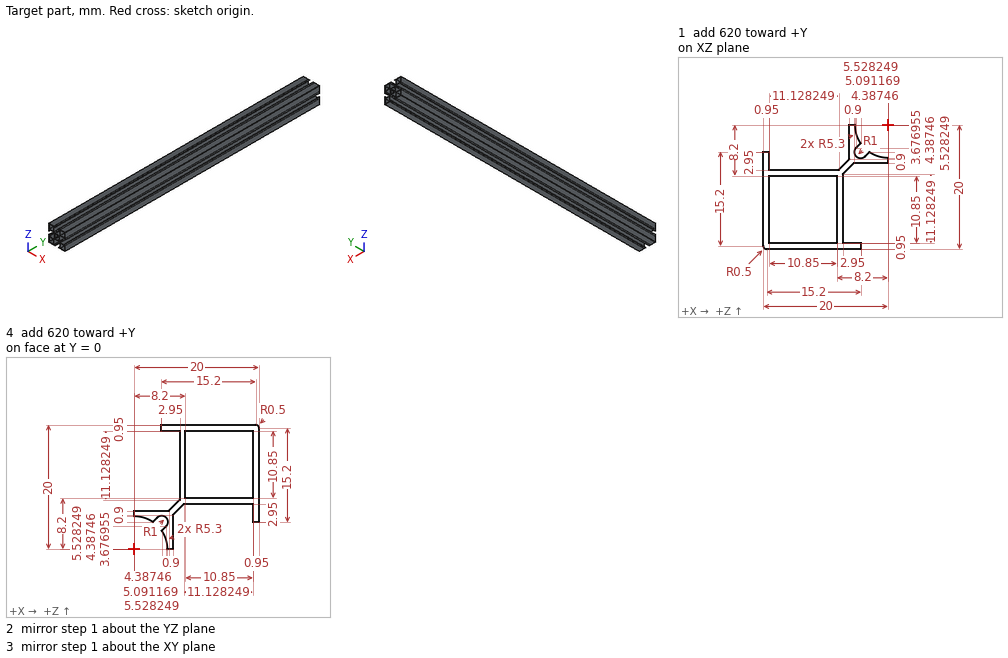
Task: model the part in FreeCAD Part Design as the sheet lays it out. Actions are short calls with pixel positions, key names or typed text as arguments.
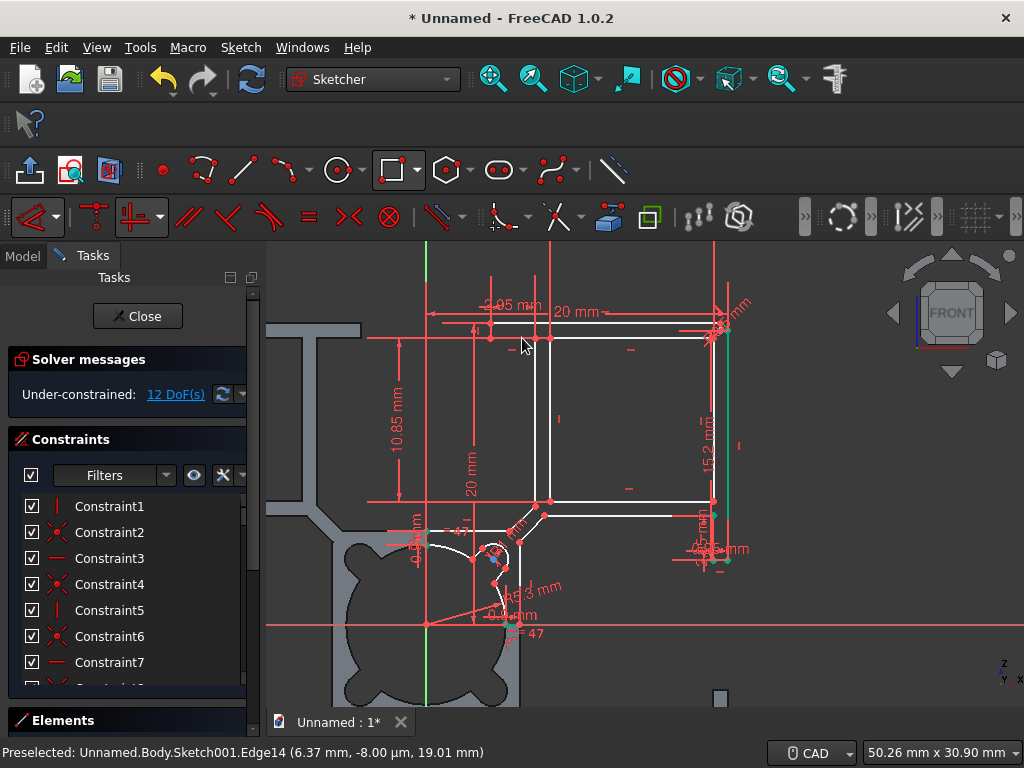
scroll(491, 331, up, 6)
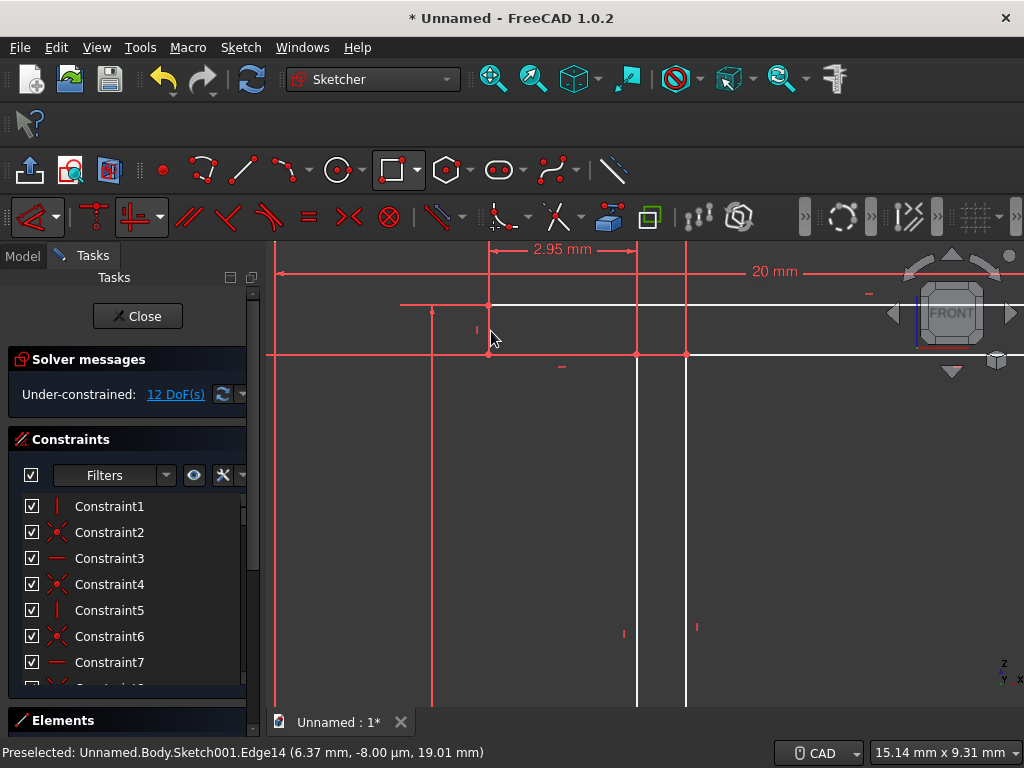
click(489, 330)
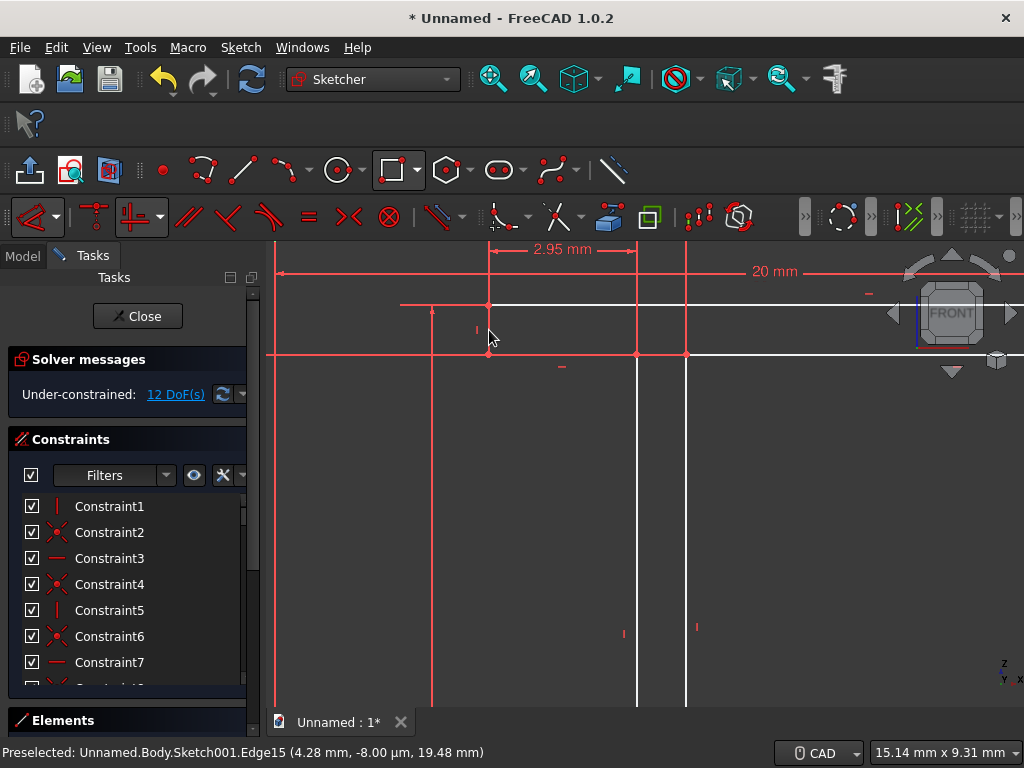
click(58, 218)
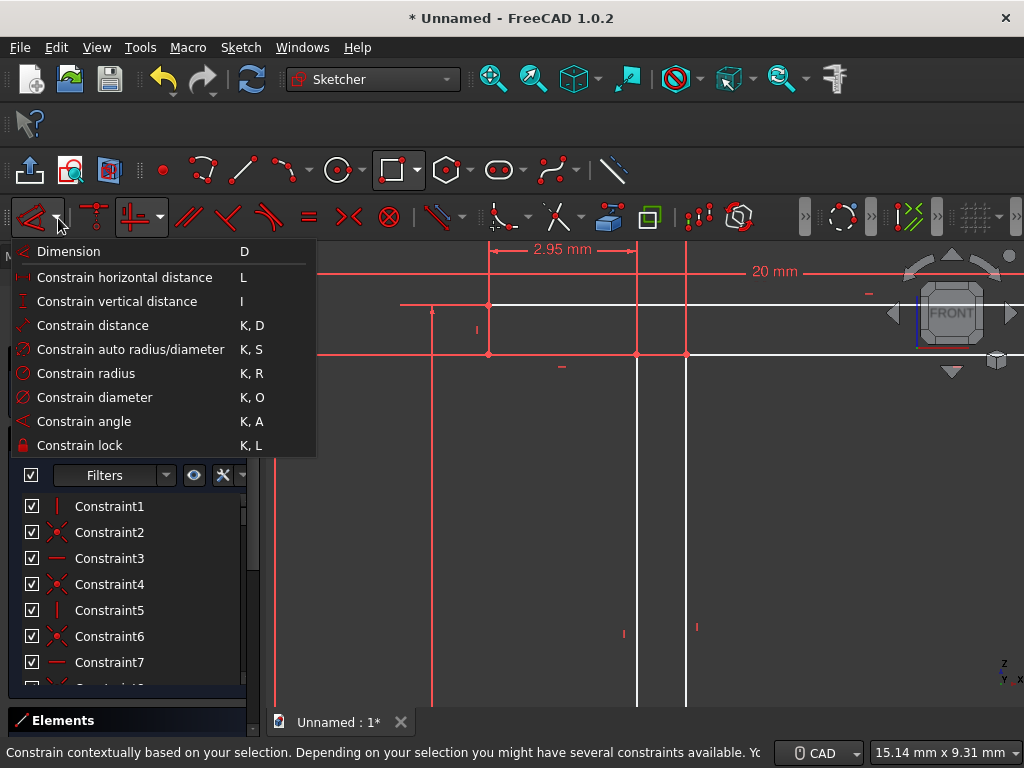
click(164, 301)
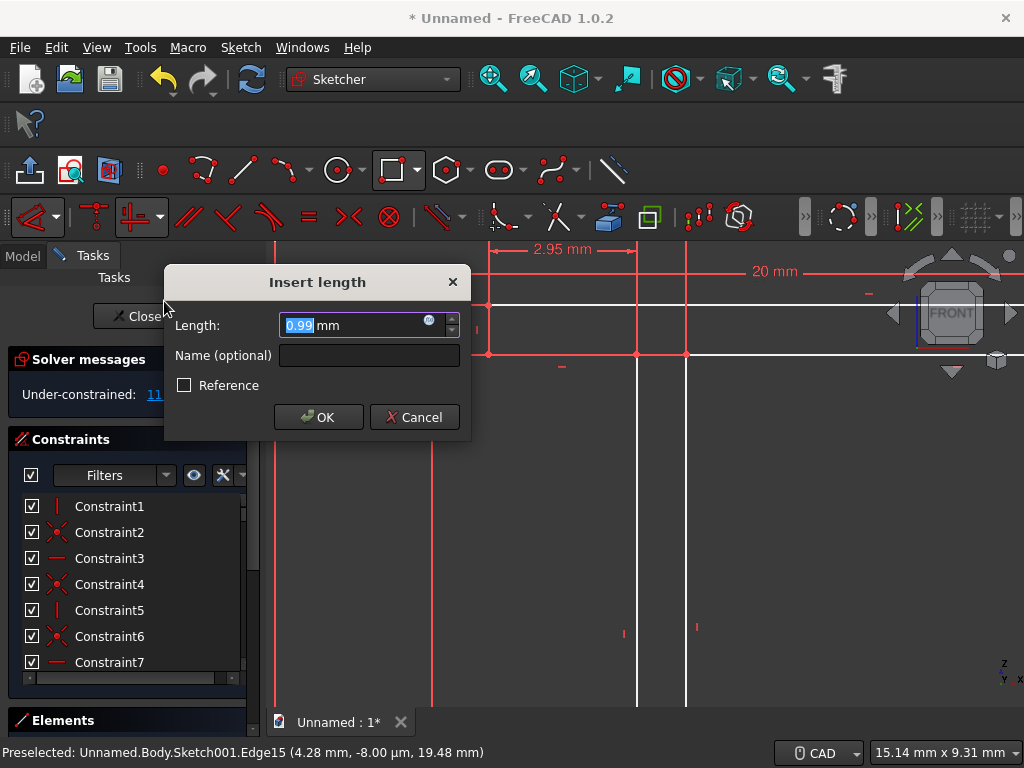
text(0.95)
key(Return)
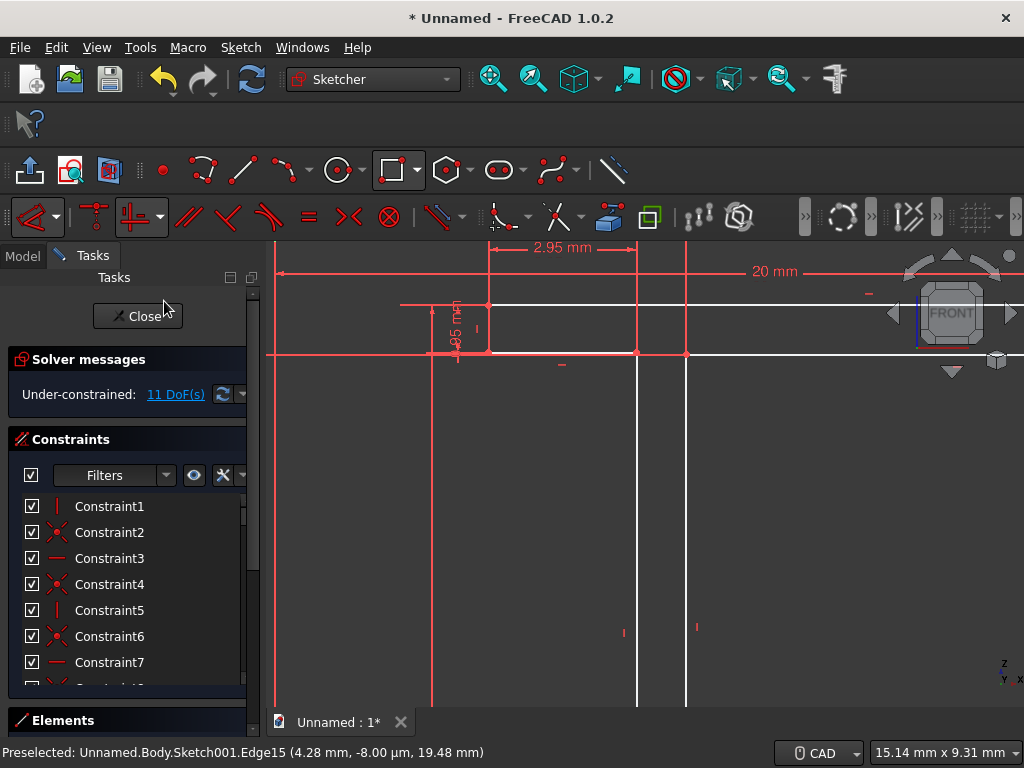
click(717, 305)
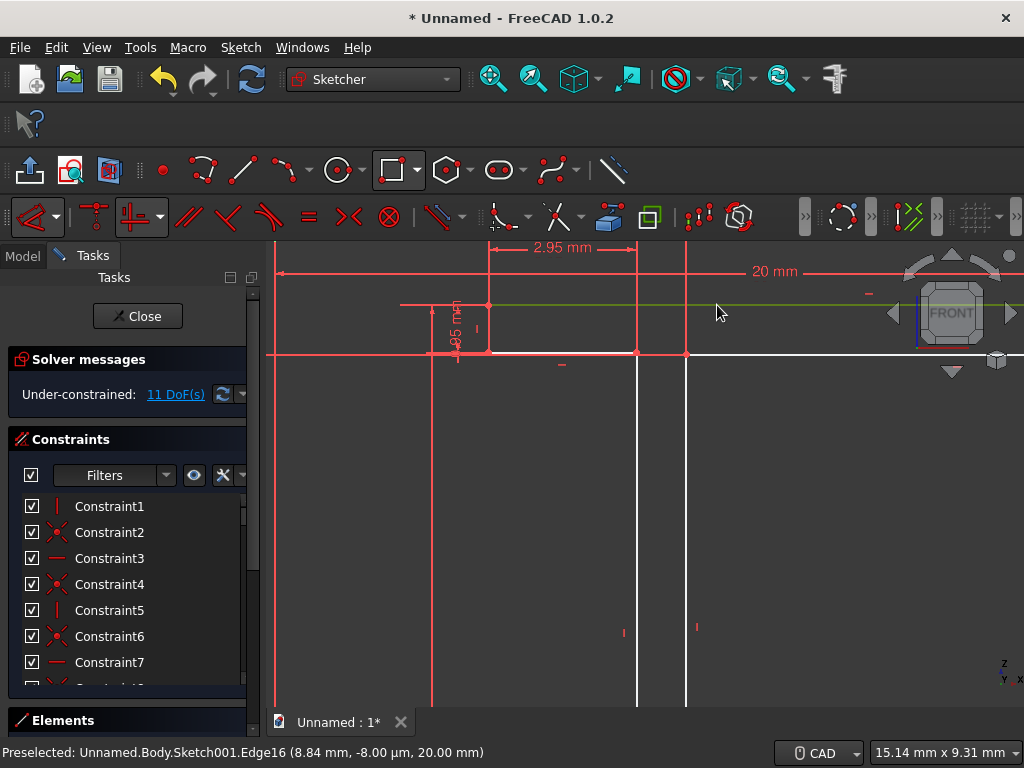
key(l)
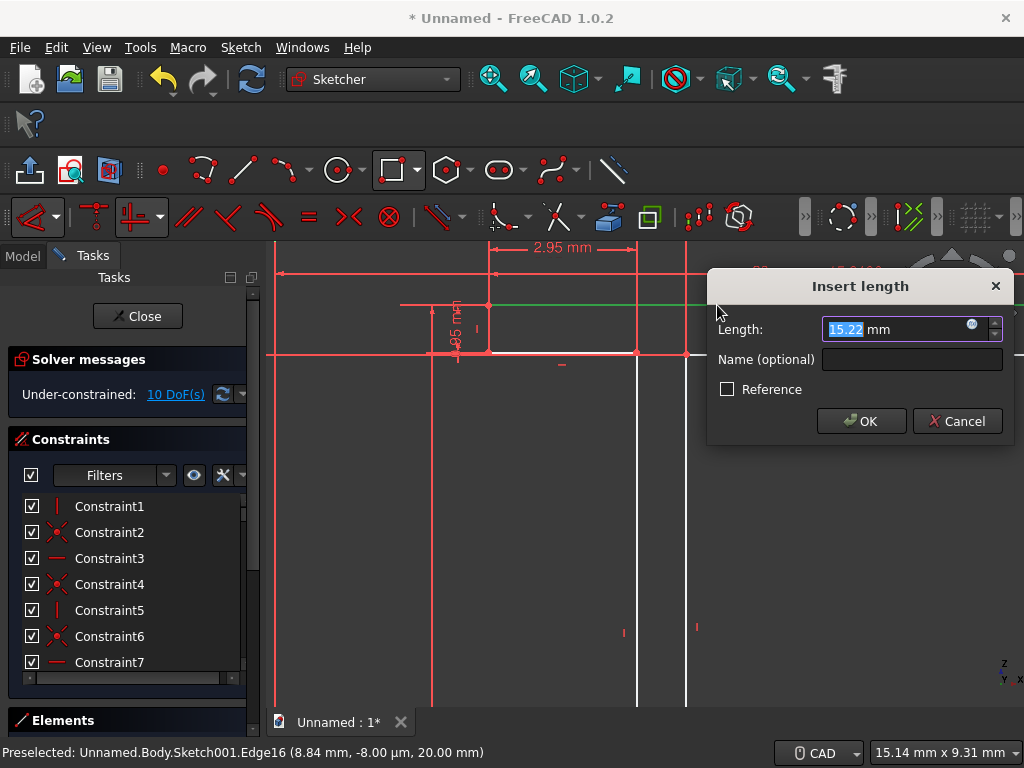
text(15.2)
key(Return)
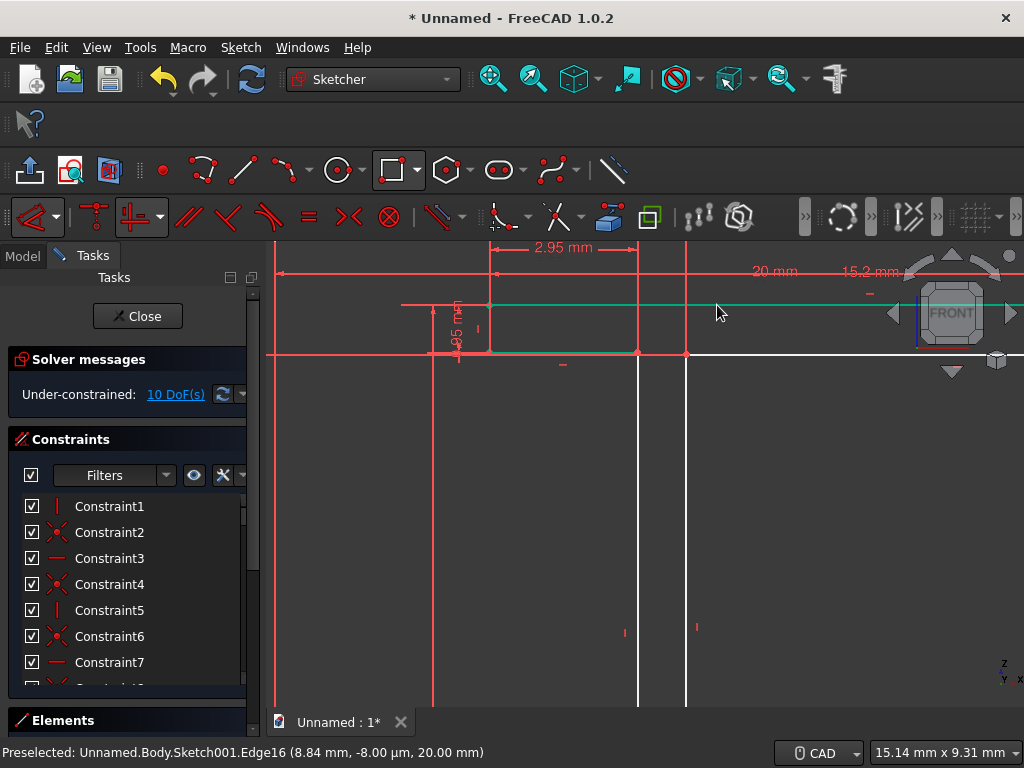
click(686, 355)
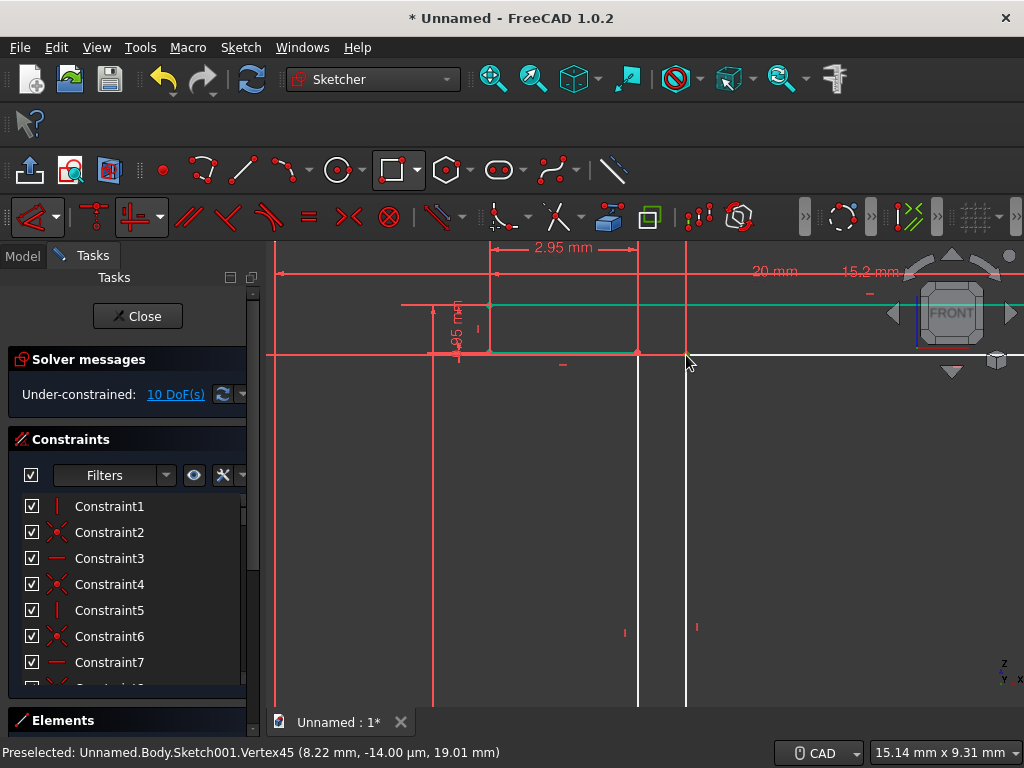
click(58, 218)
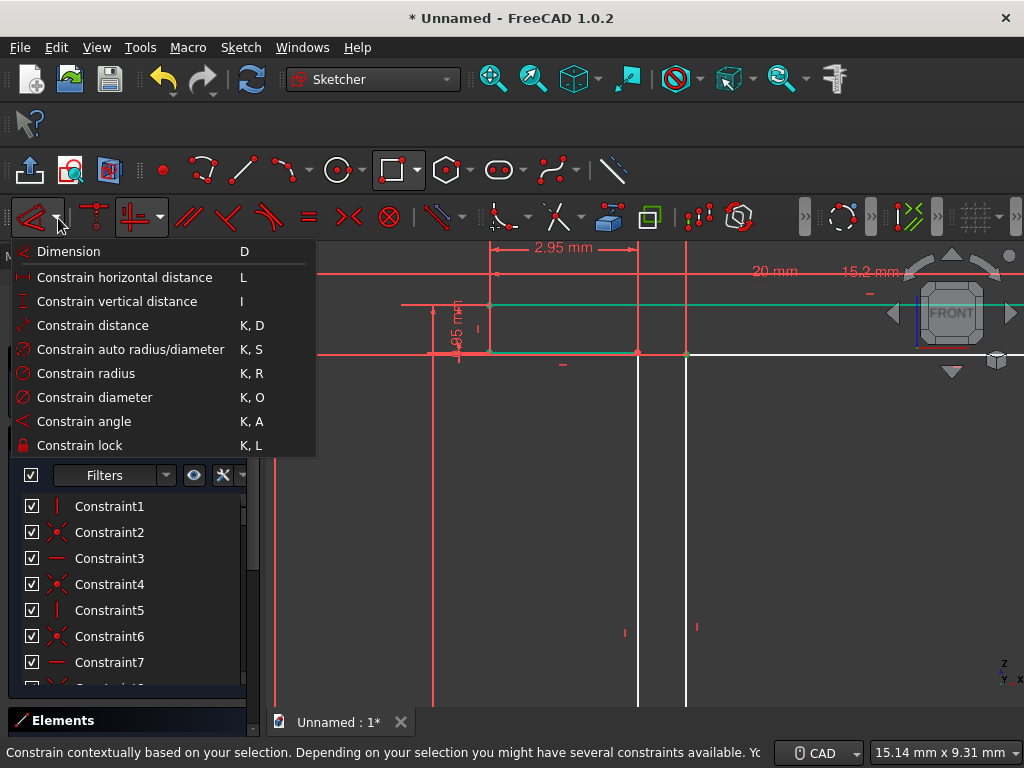
click(164, 277)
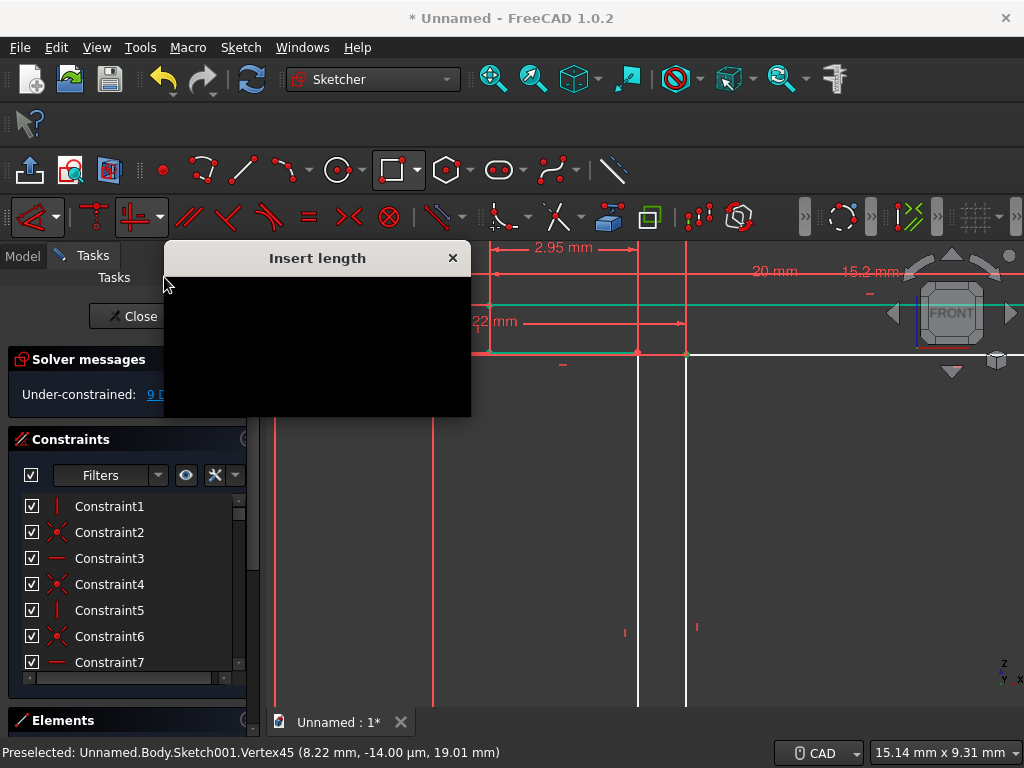
text(8.2)
key(Return)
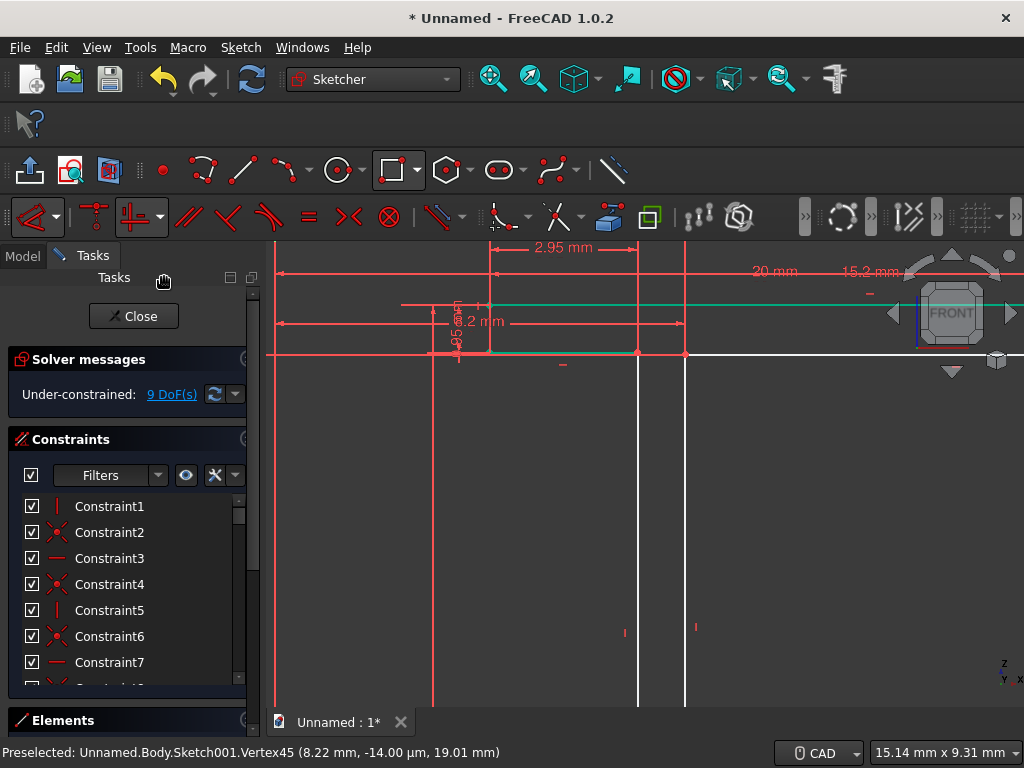
scroll(491, 331, down, 6)